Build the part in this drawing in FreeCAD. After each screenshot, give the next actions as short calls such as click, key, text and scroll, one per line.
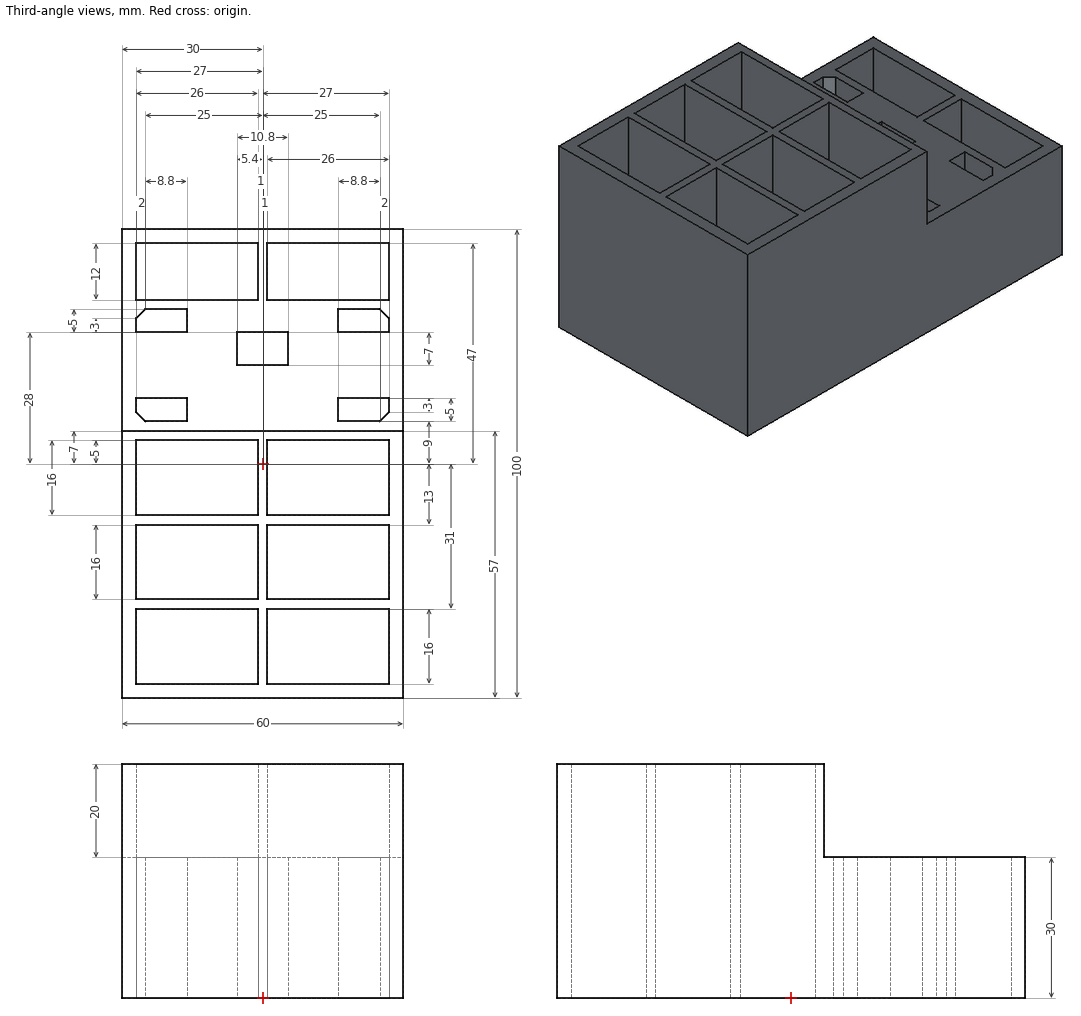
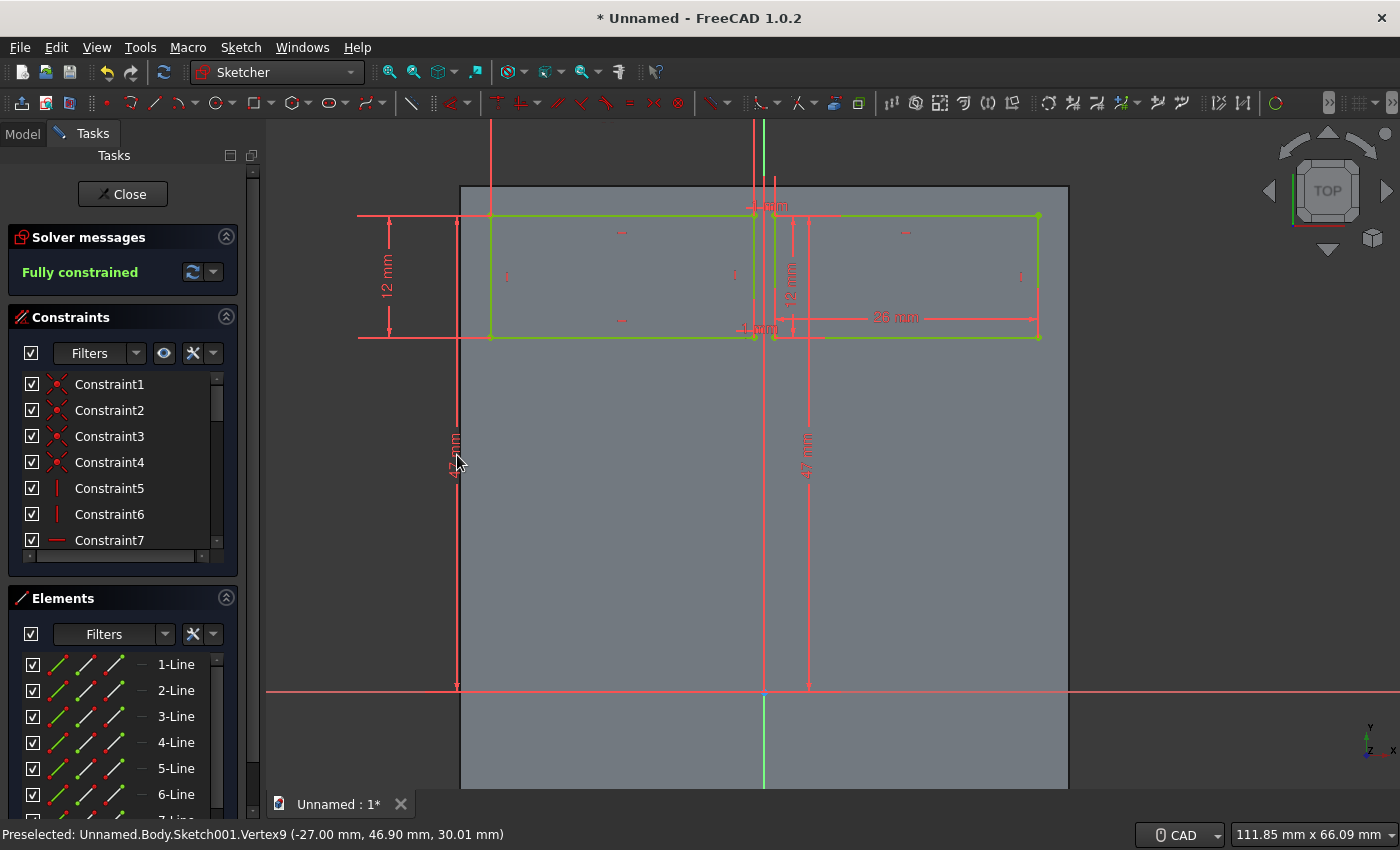
click(123, 194)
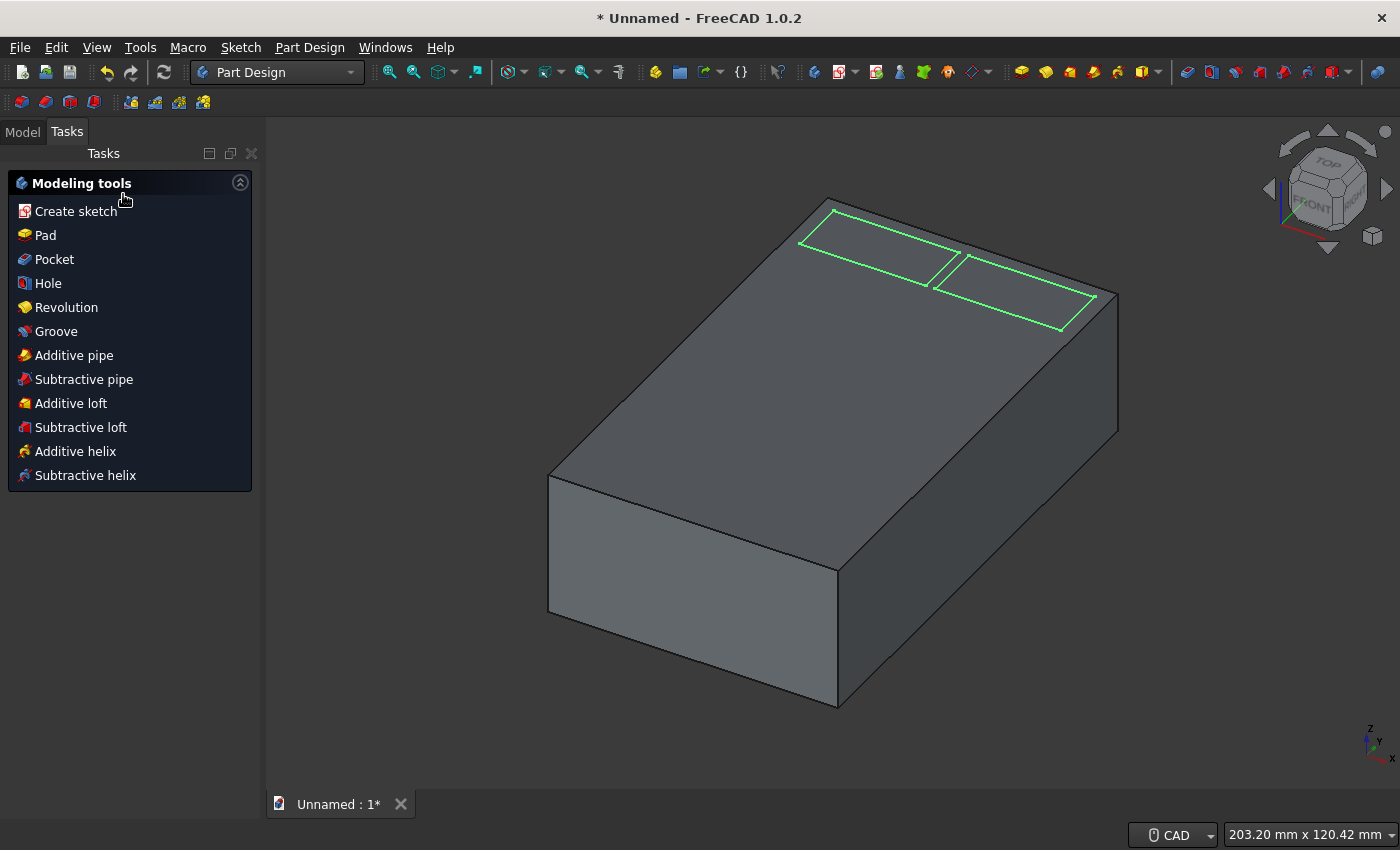
click(1188, 72)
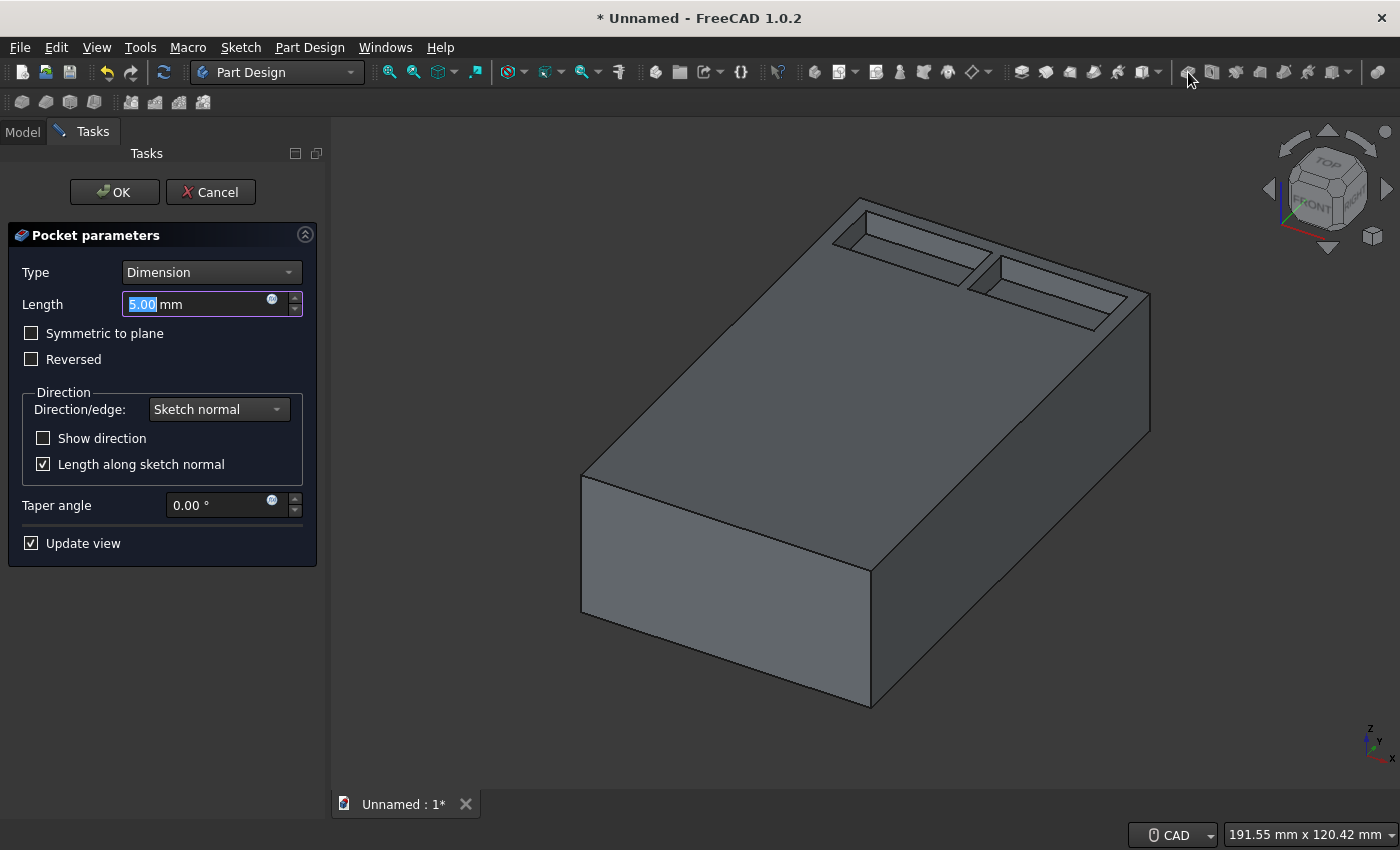
click(212, 272)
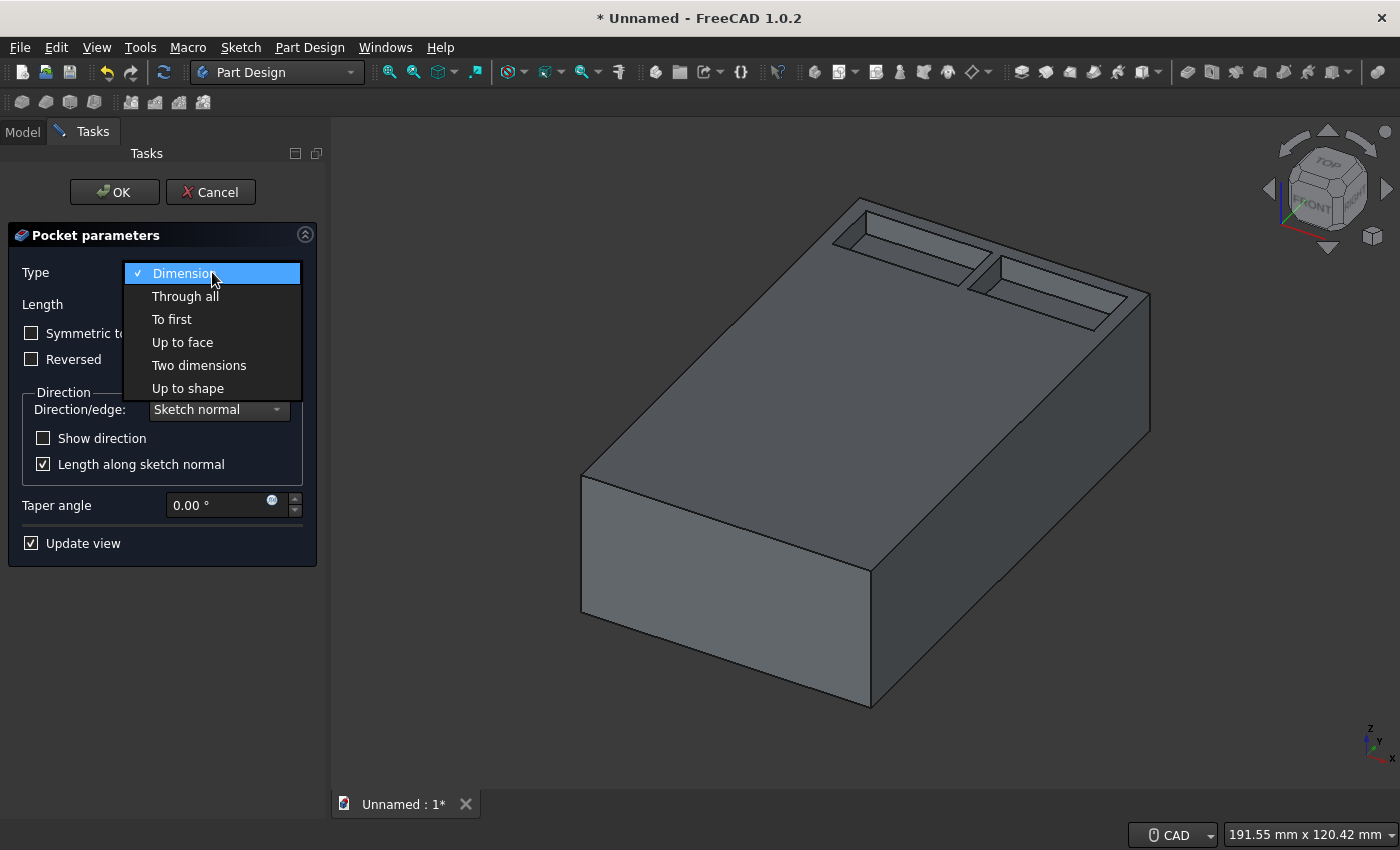
click(212, 296)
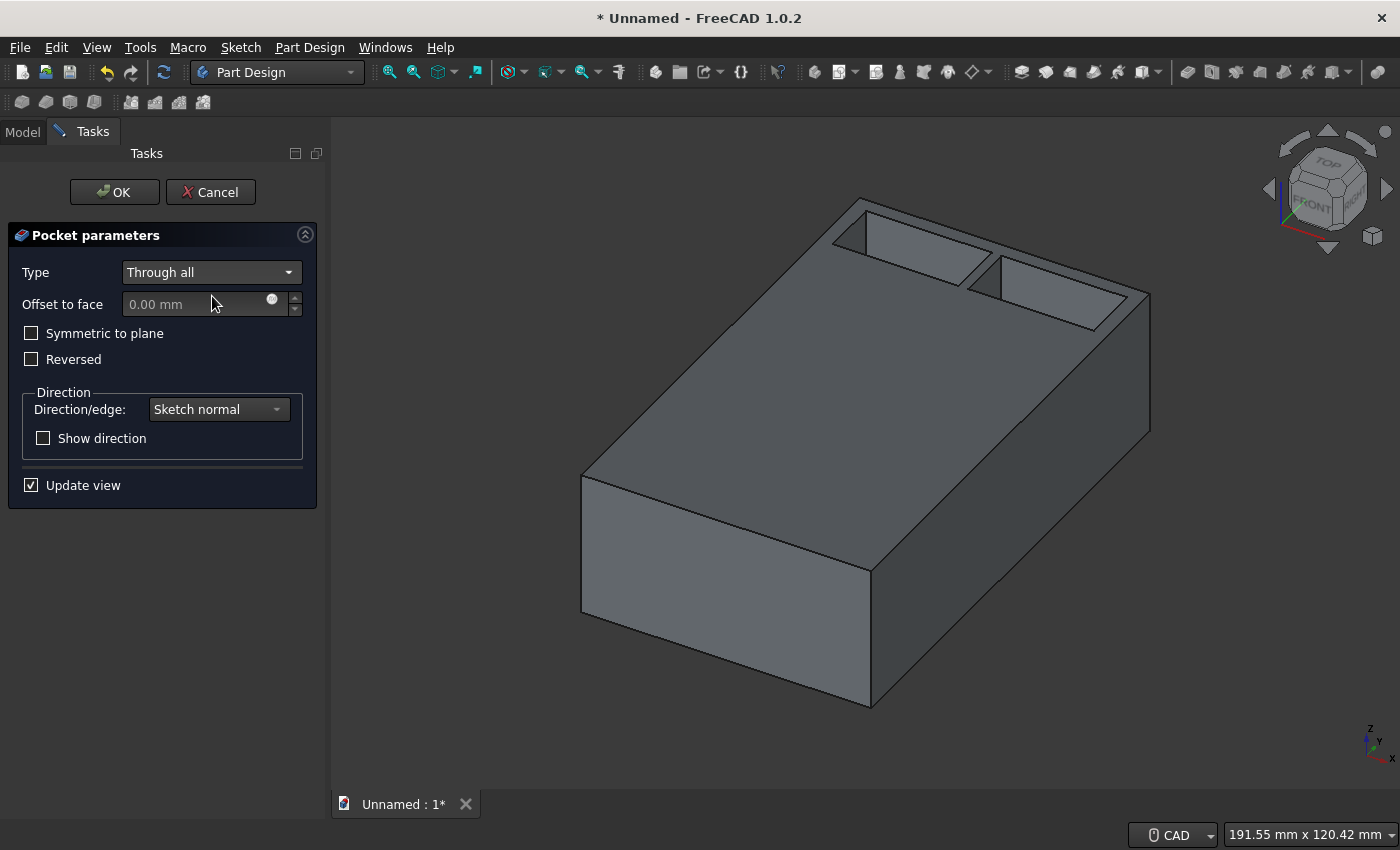
click(115, 192)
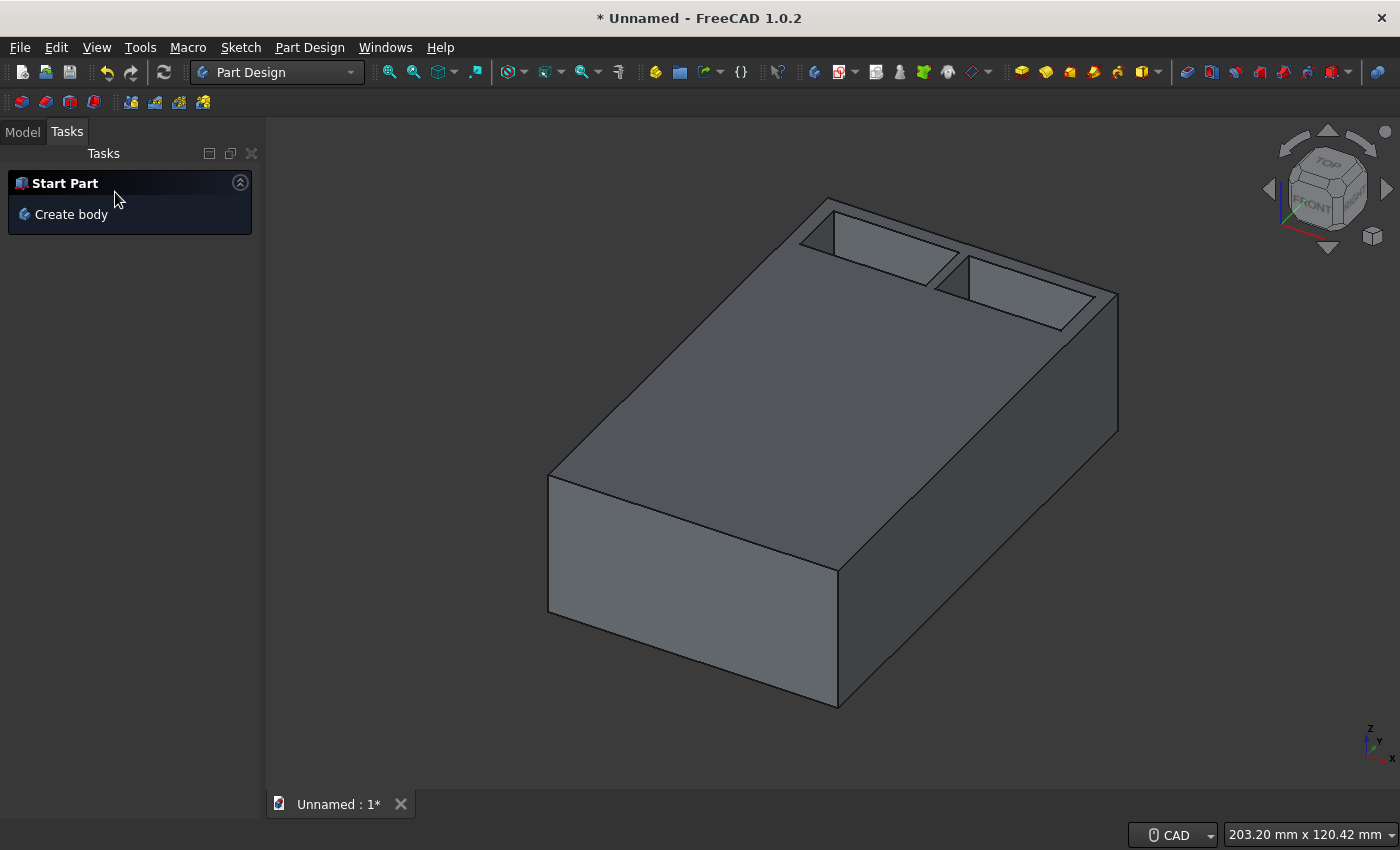
click(833, 383)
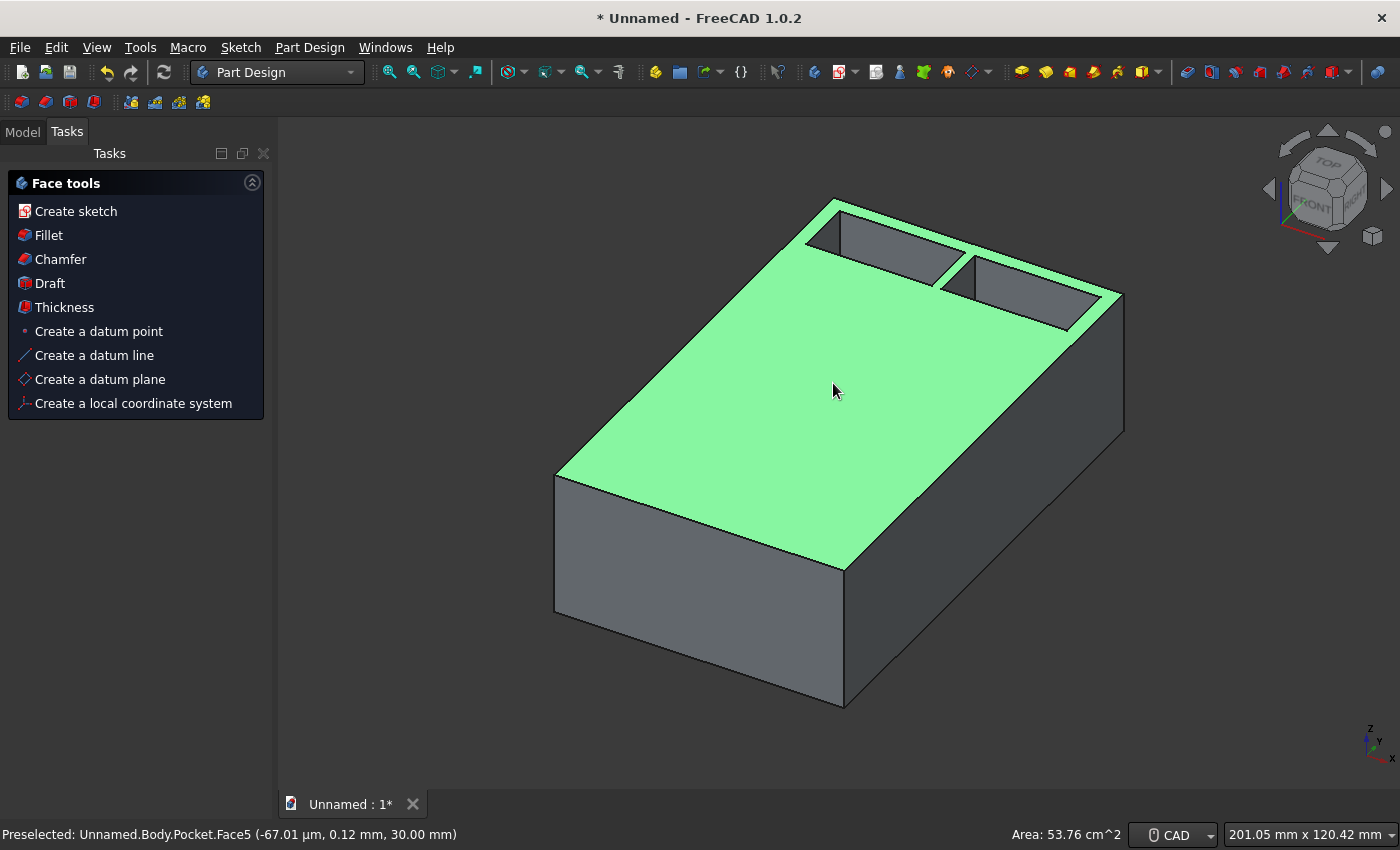
click(840, 72)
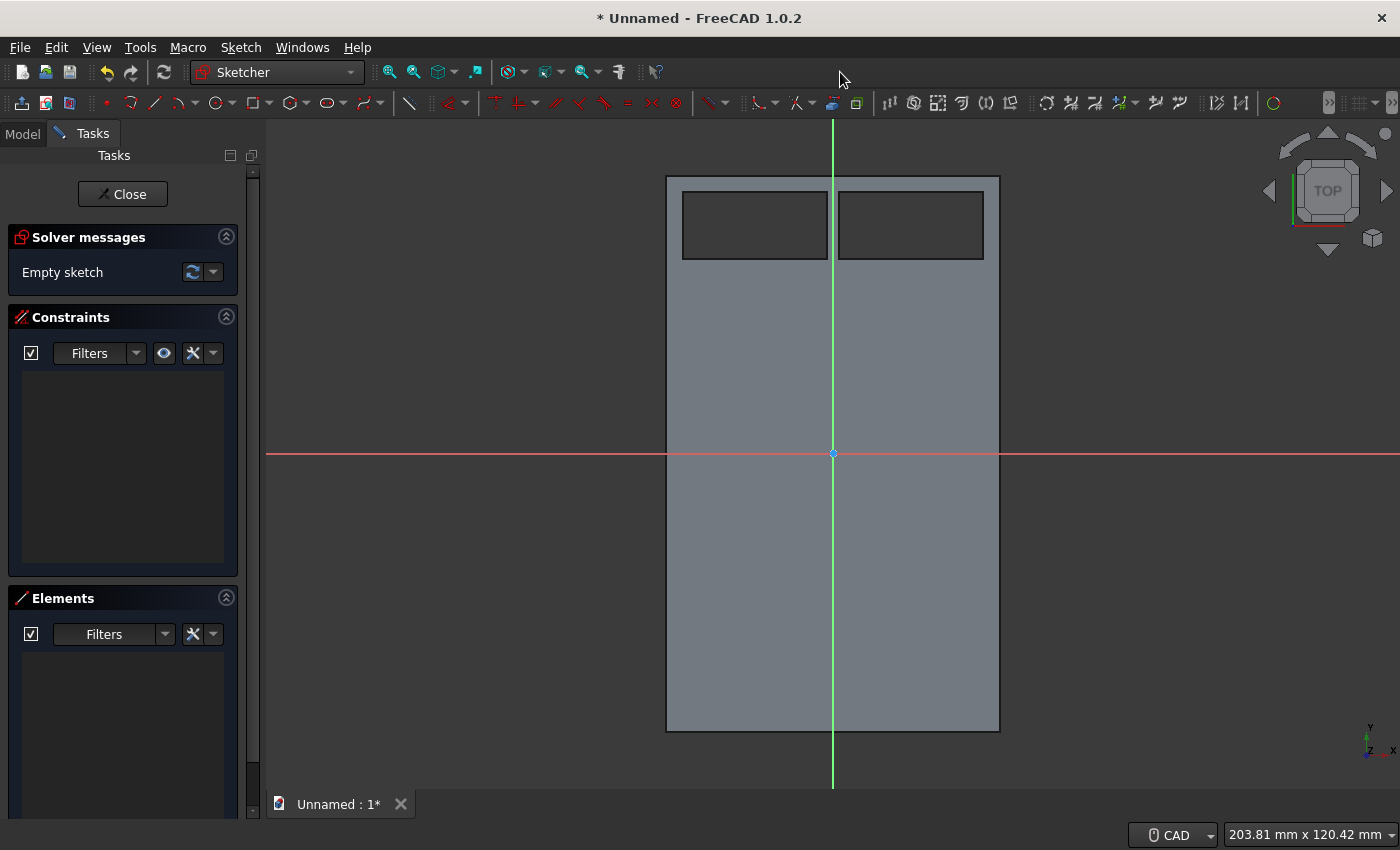
scroll(972, 761, up, 2)